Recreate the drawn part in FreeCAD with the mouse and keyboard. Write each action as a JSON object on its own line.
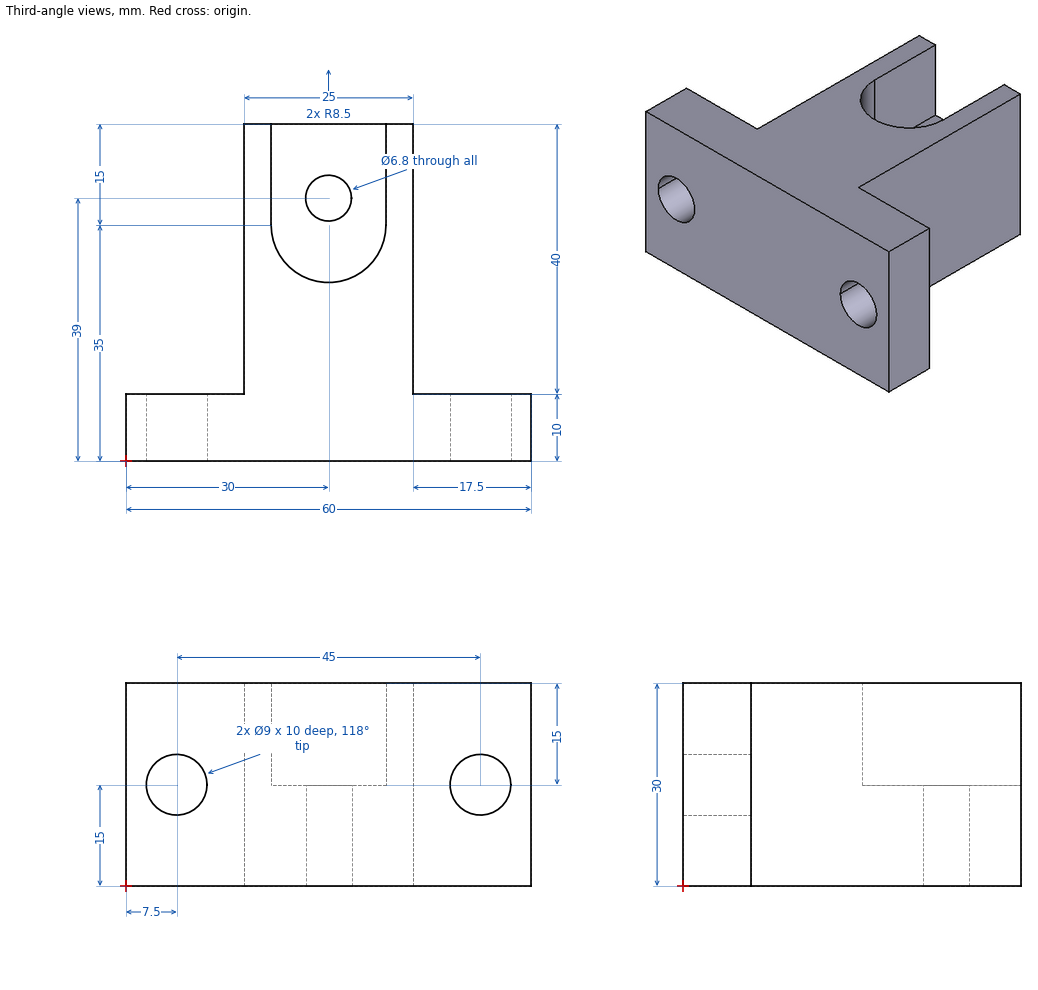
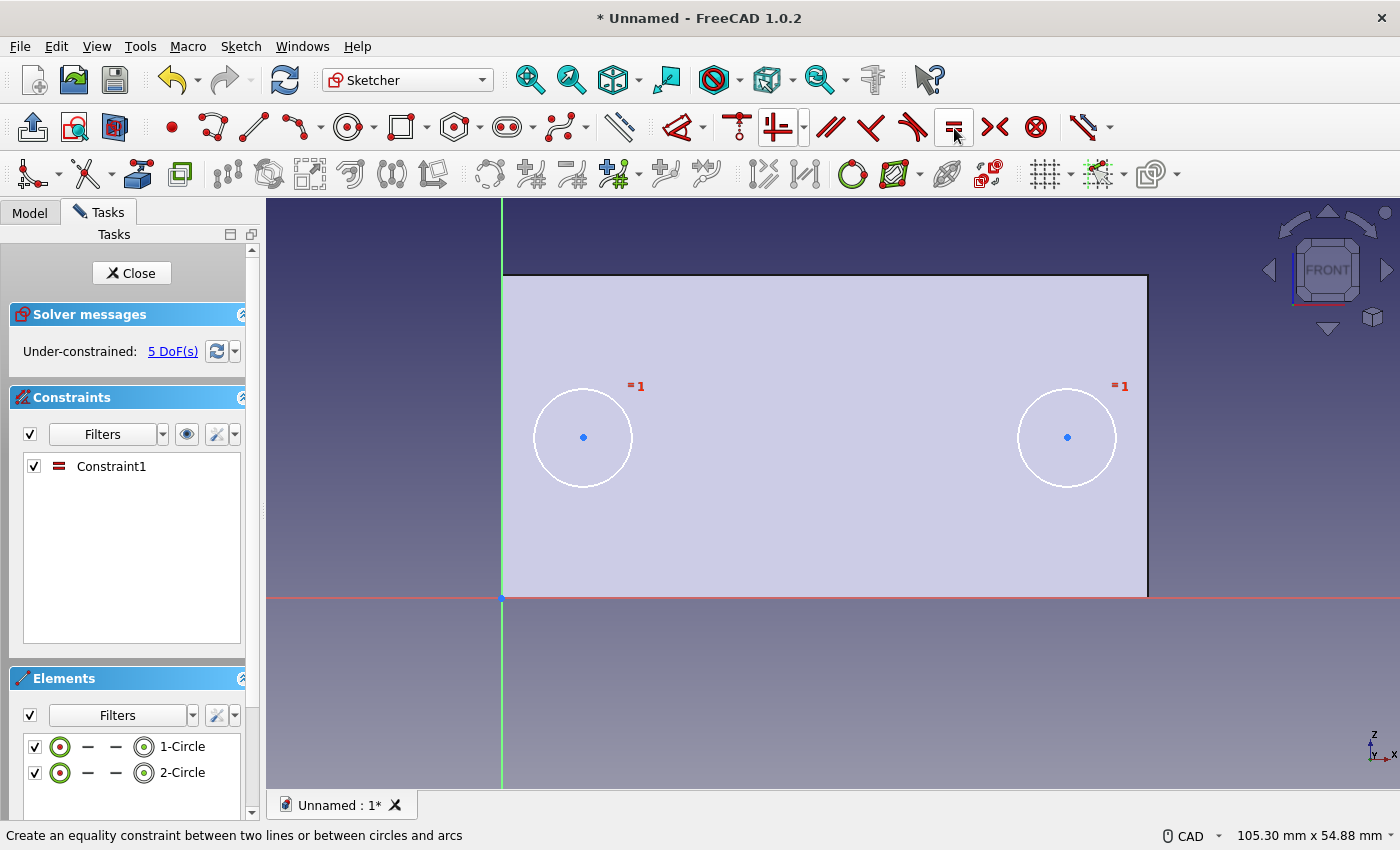
{"action": "left_click", "coordinate": [583, 438]}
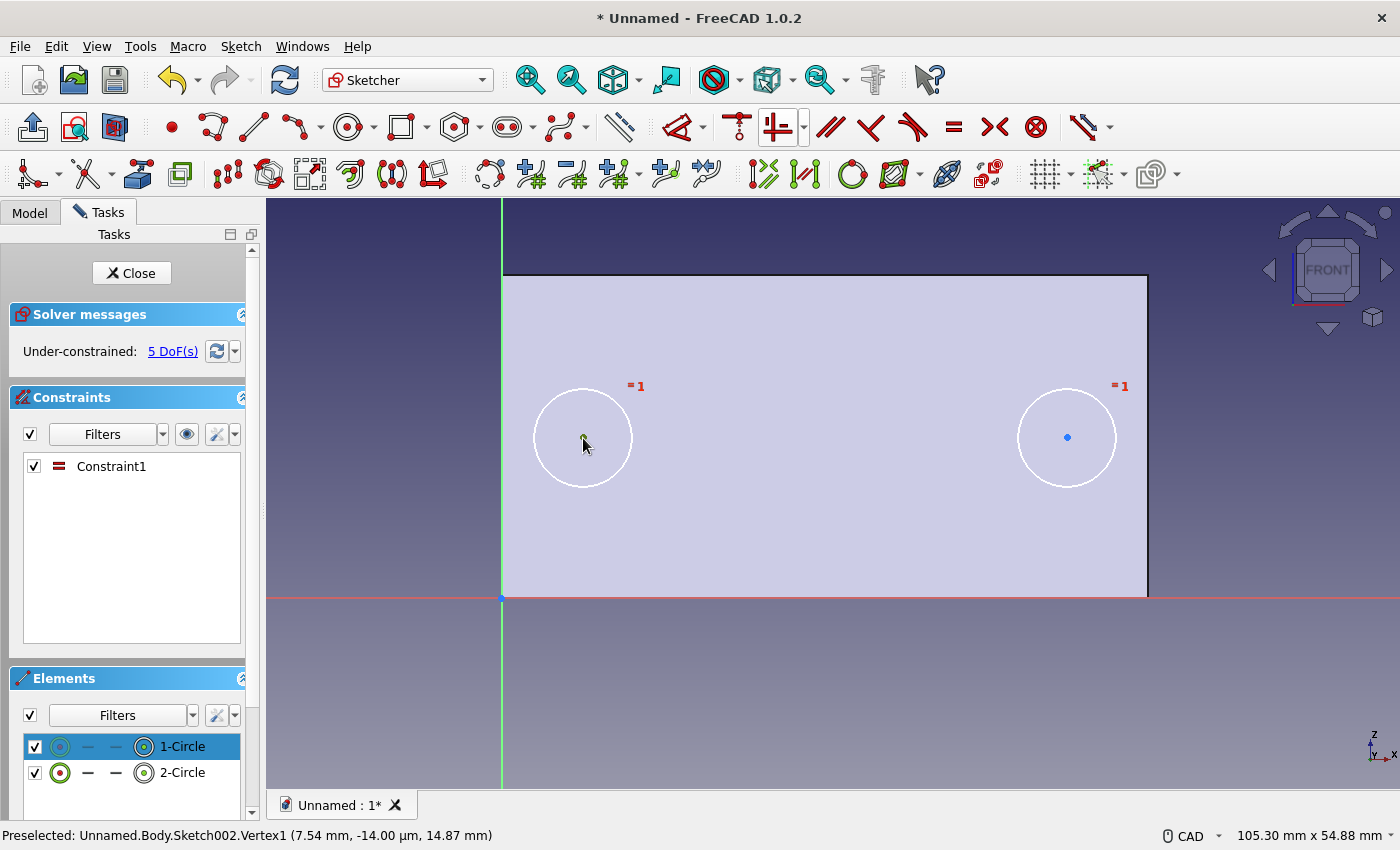
{"action": "left_click", "coordinate": [1067, 438]}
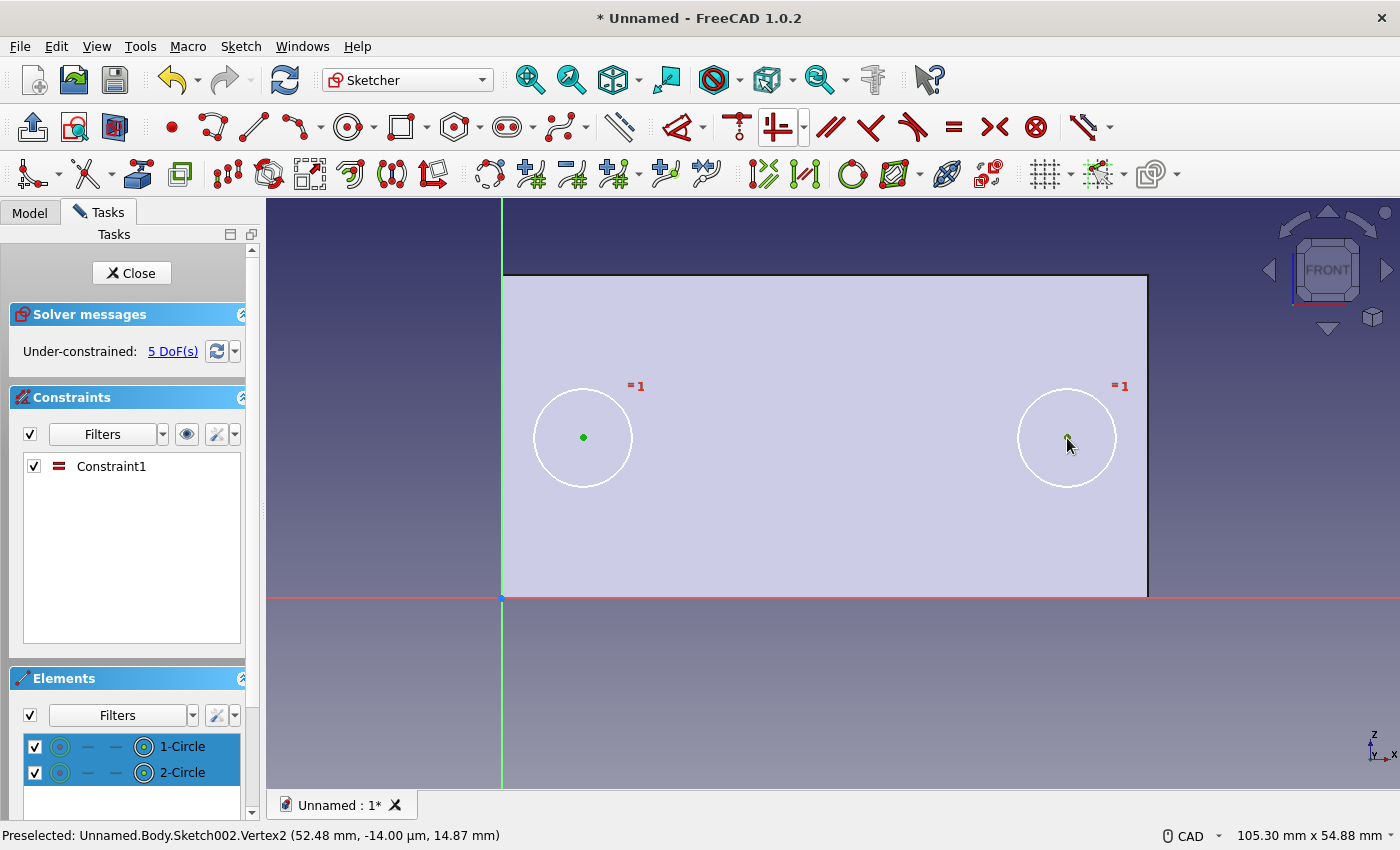
{"action": "key", "text": "h"}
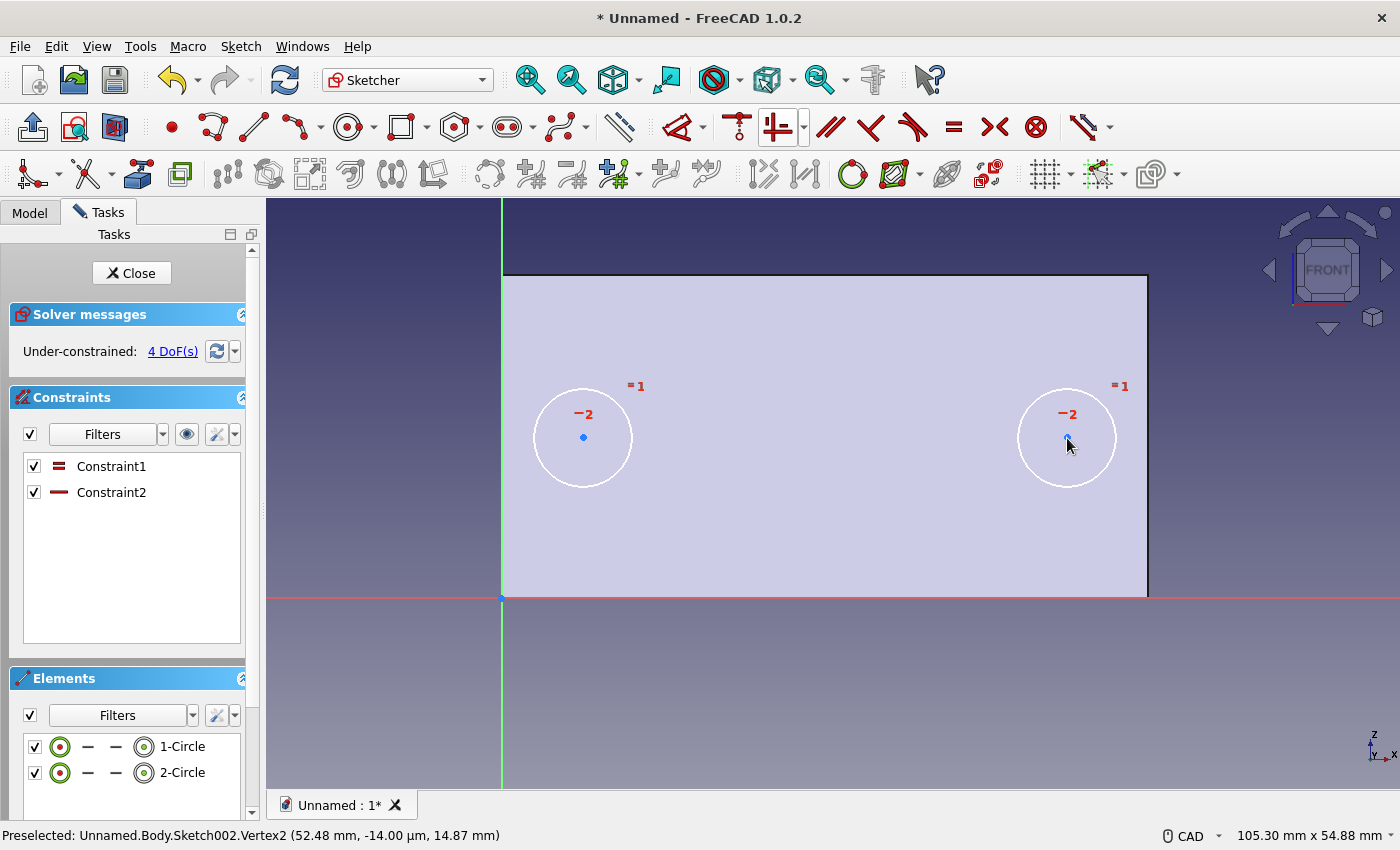
{"action": "left_click", "coordinate": [676, 128]}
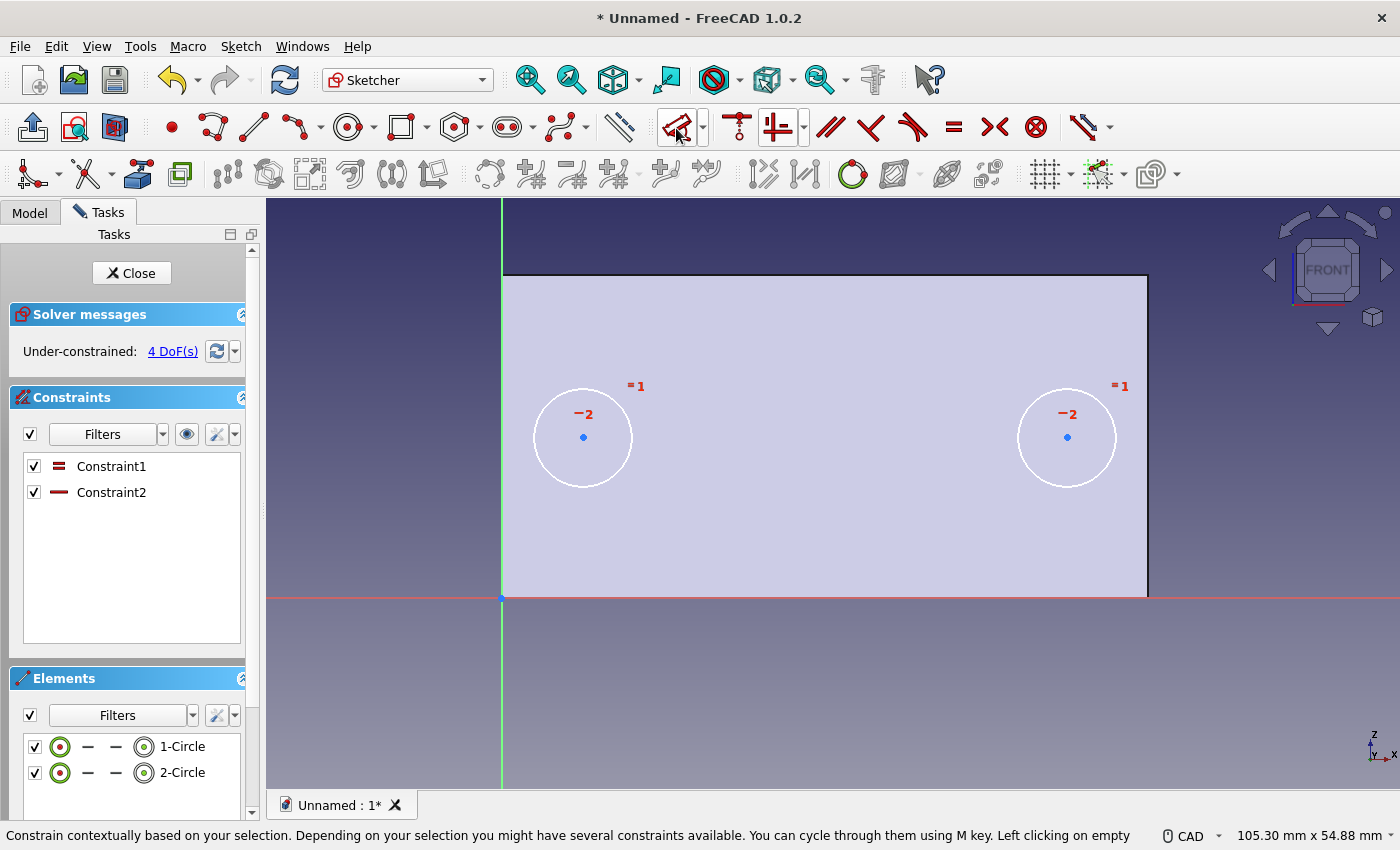
{"action": "left_click", "coordinate": [617, 403]}
{"action": "left_click", "coordinate": [639, 380]}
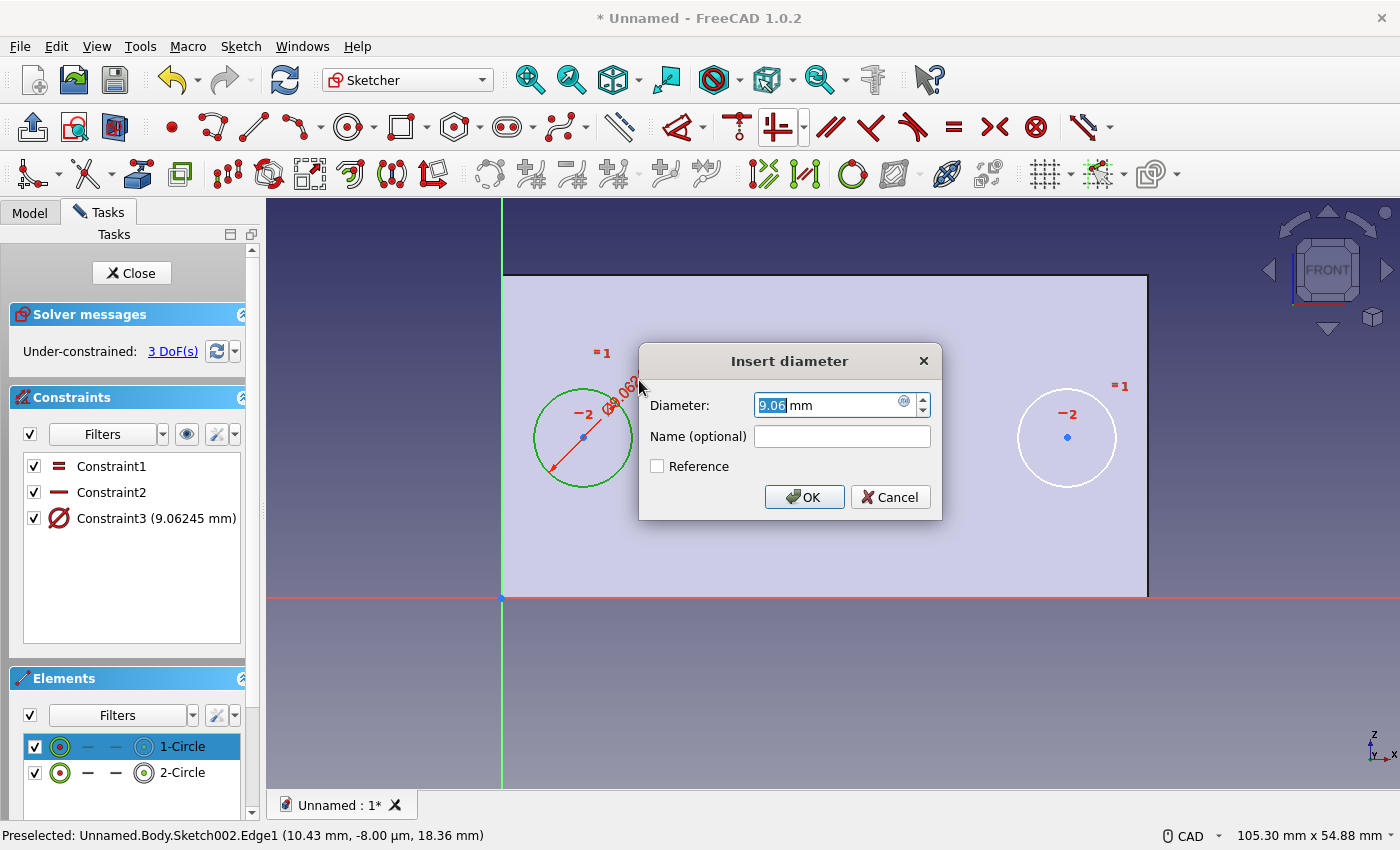
{"action": "type", "text": "9"}
{"action": "key", "text": "Return"}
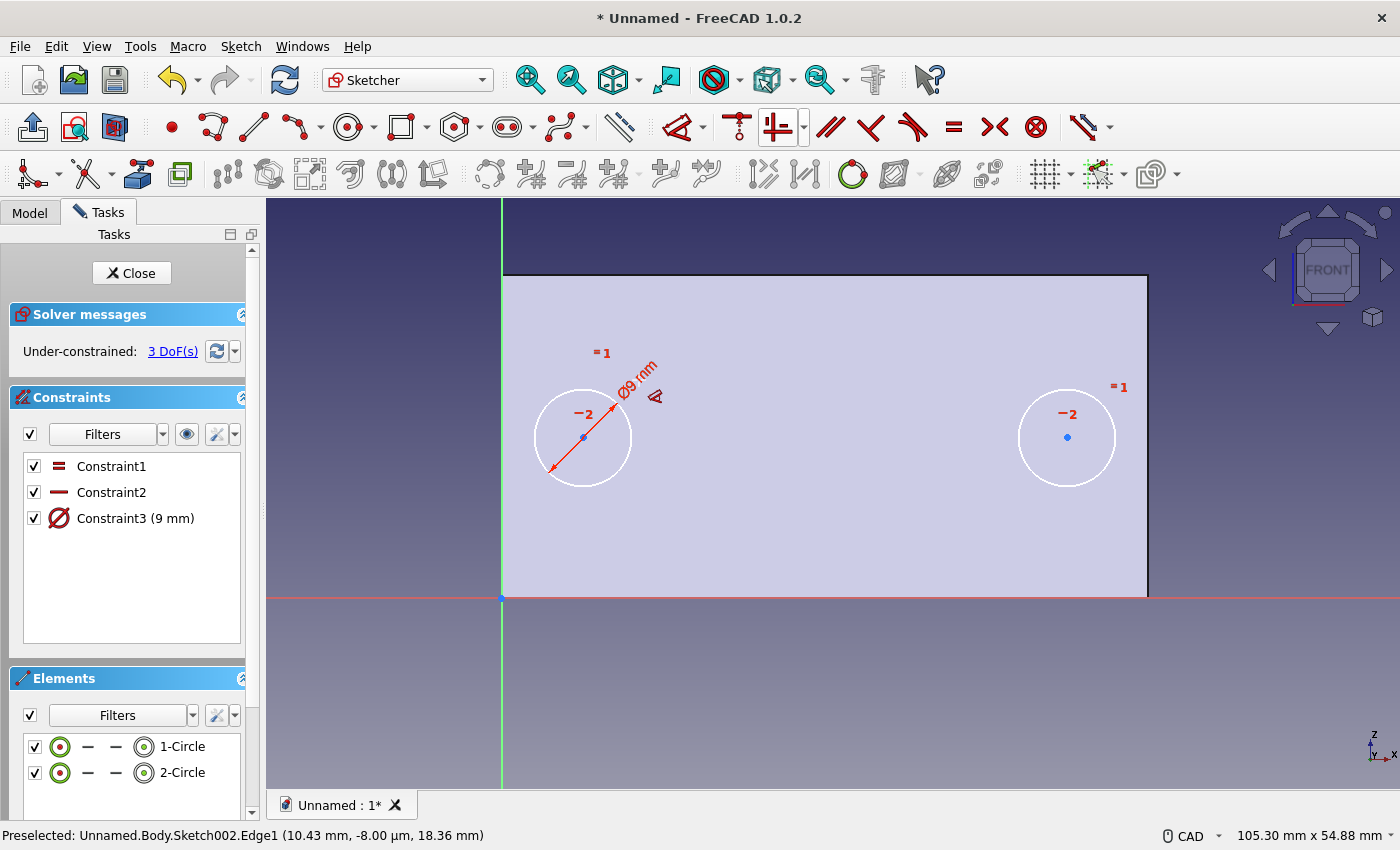
{"action": "left_click", "coordinate": [583, 438]}
{"action": "left_click", "coordinate": [468, 518]}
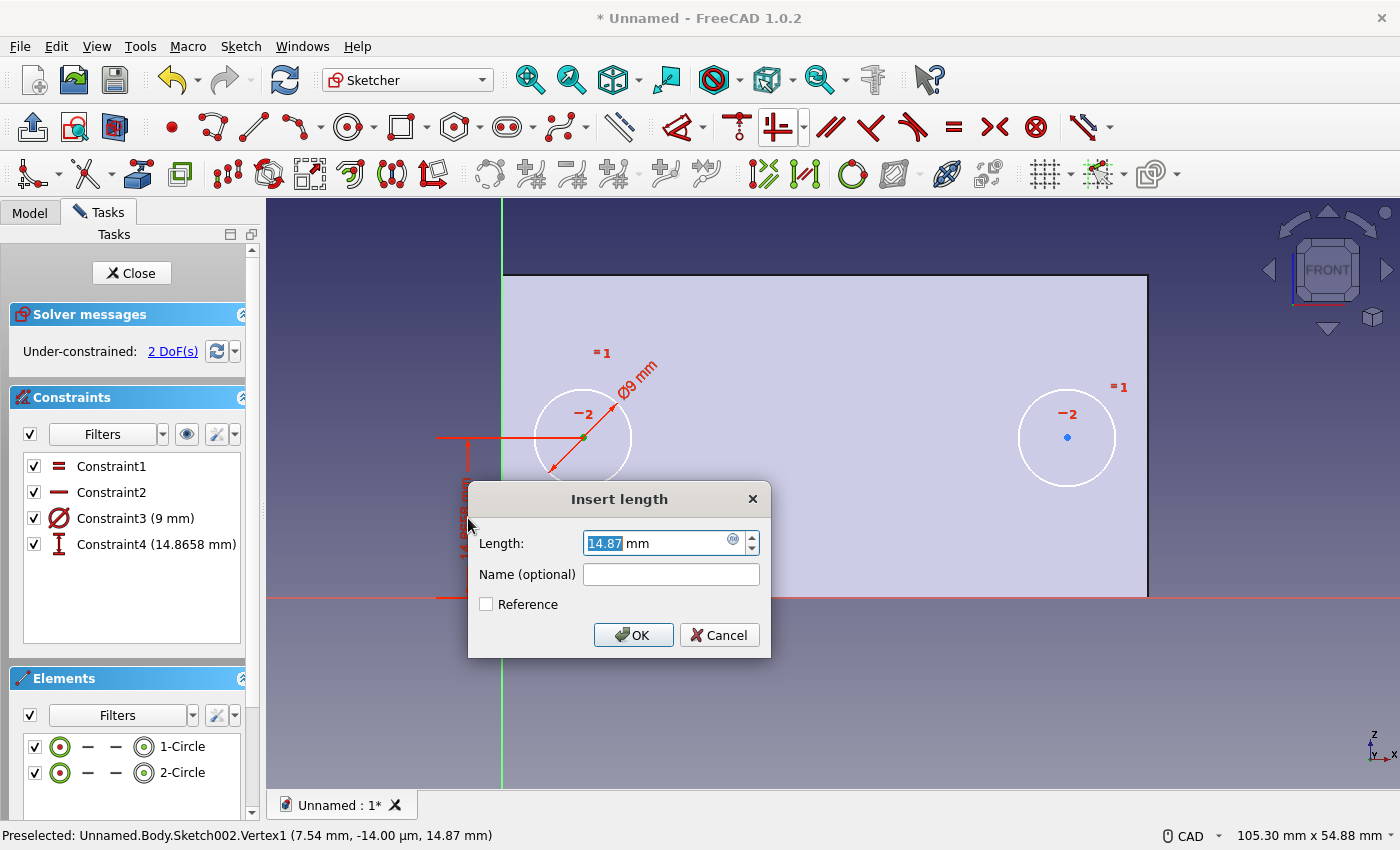
{"action": "type", "text": "15"}
{"action": "key", "text": "Return"}